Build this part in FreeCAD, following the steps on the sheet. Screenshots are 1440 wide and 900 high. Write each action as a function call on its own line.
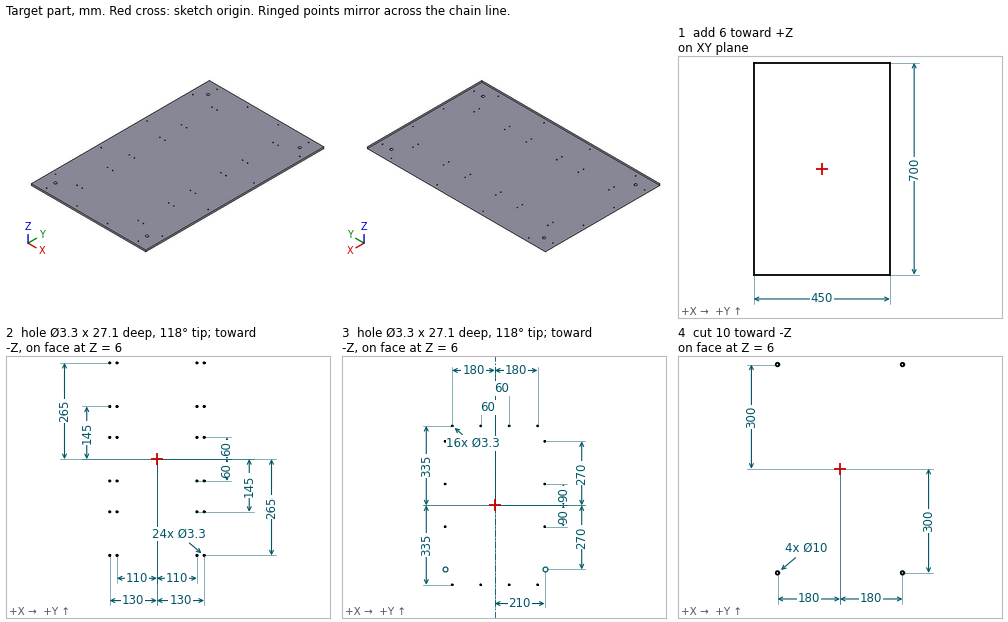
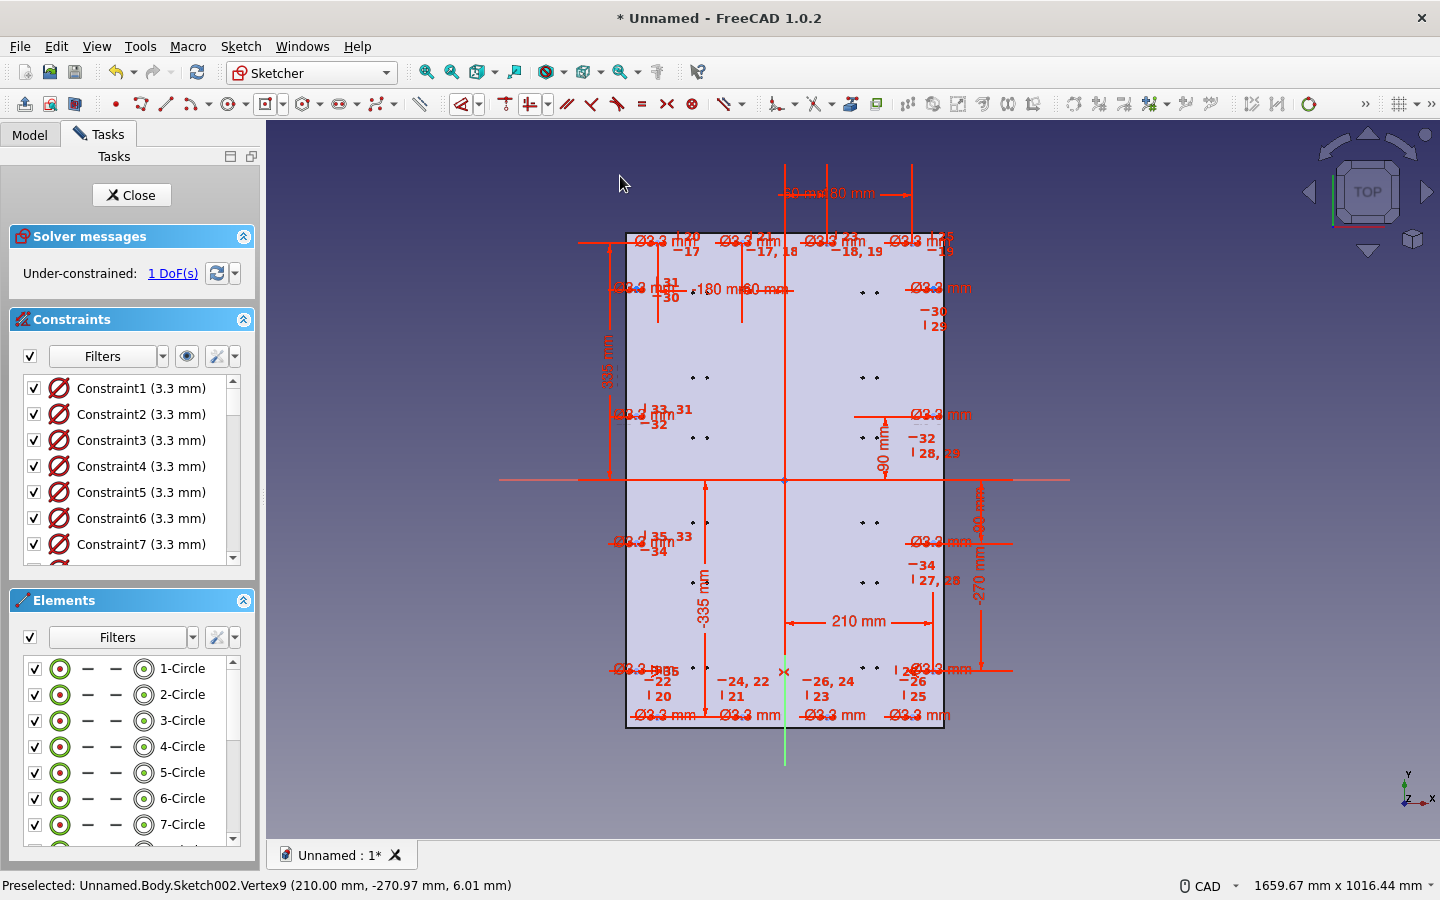
click(933, 290)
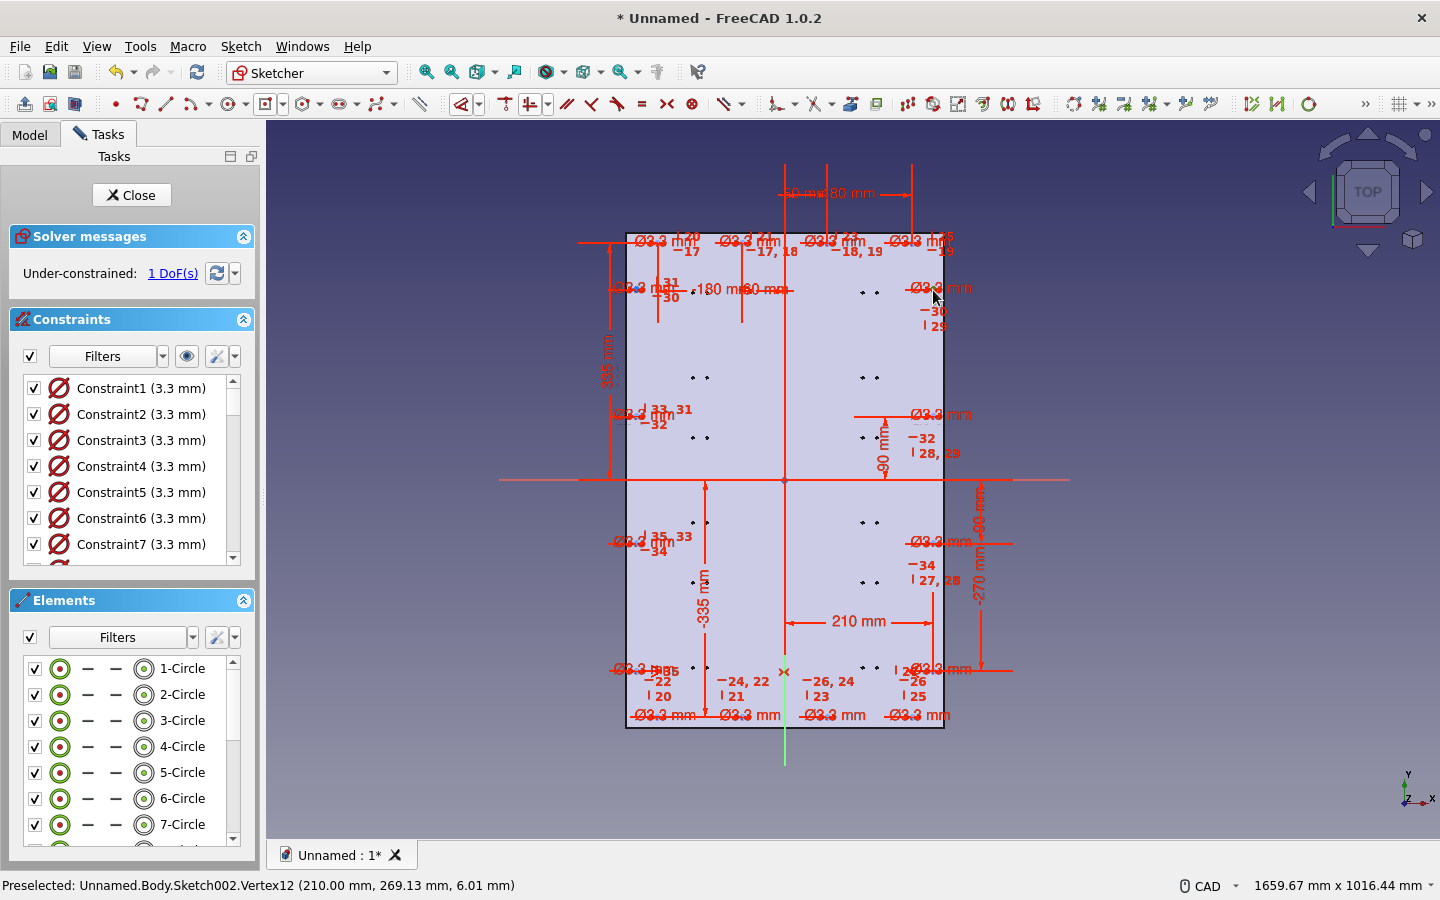
key(i)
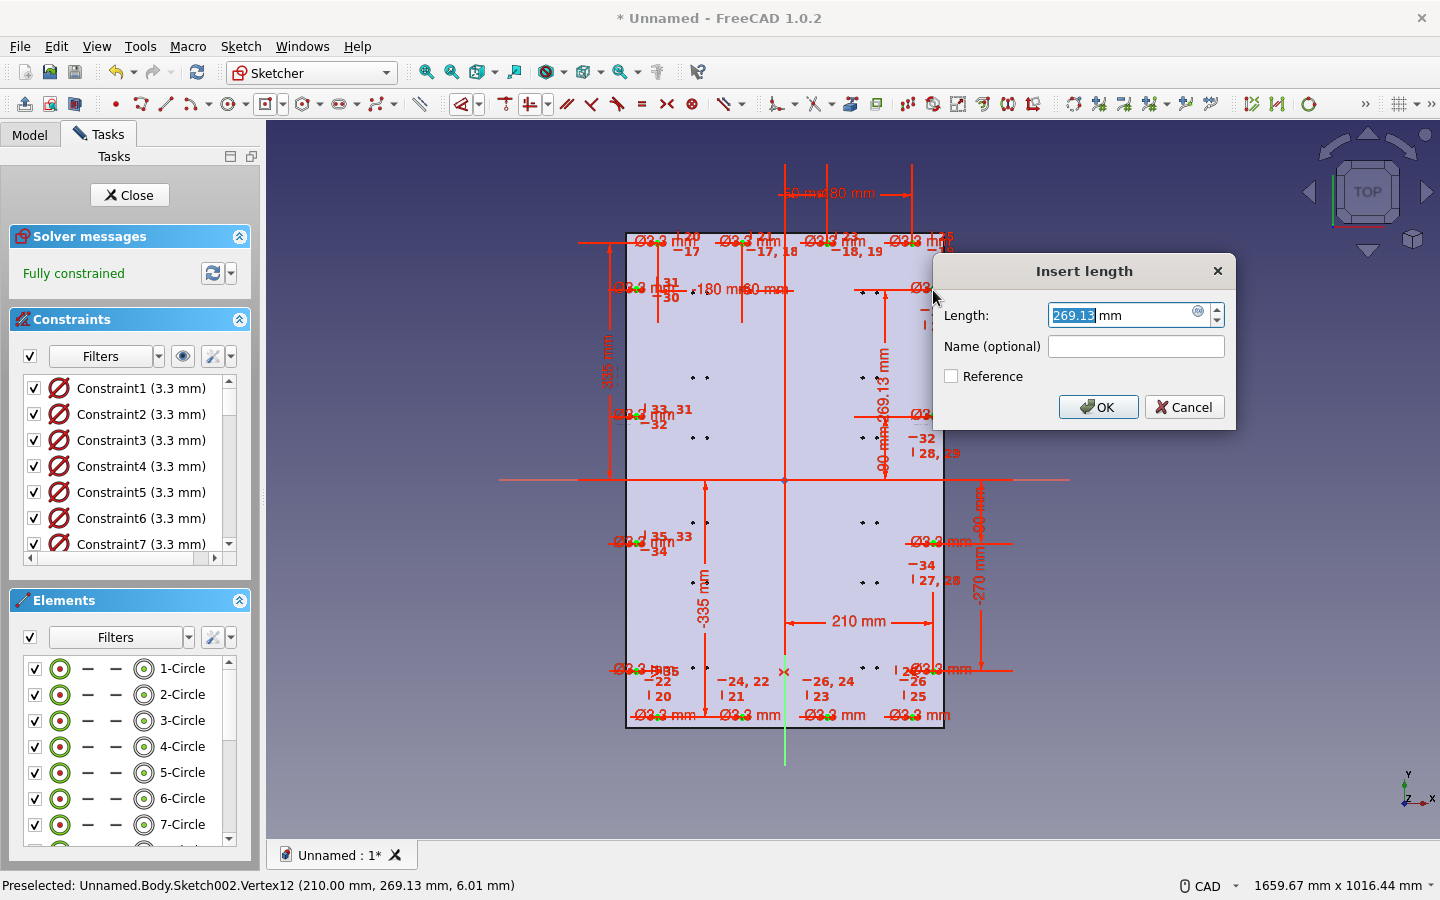
text(270)
key(Return)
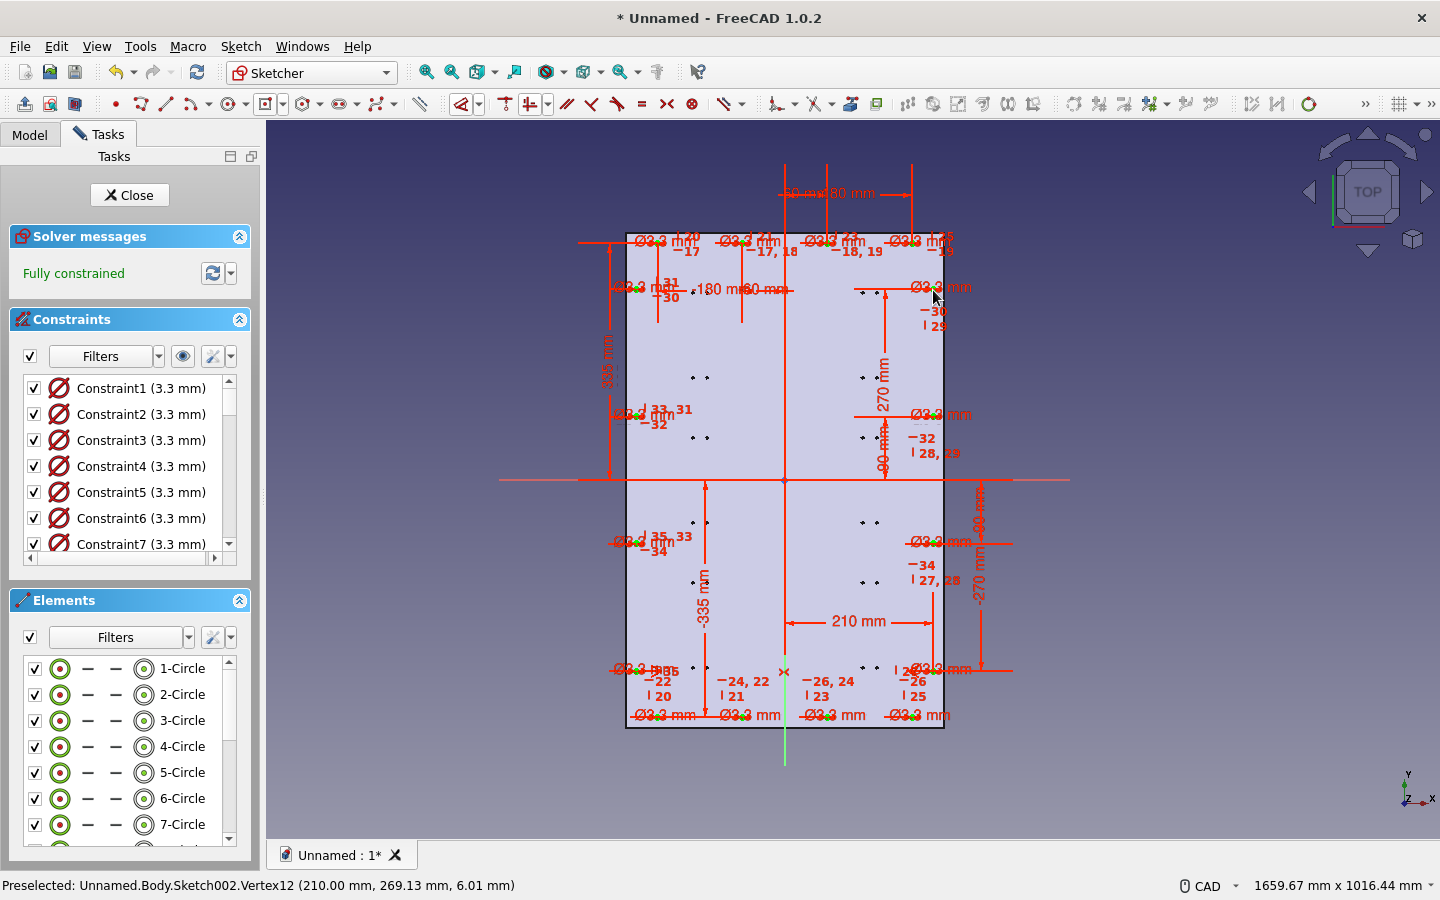
click(130, 195)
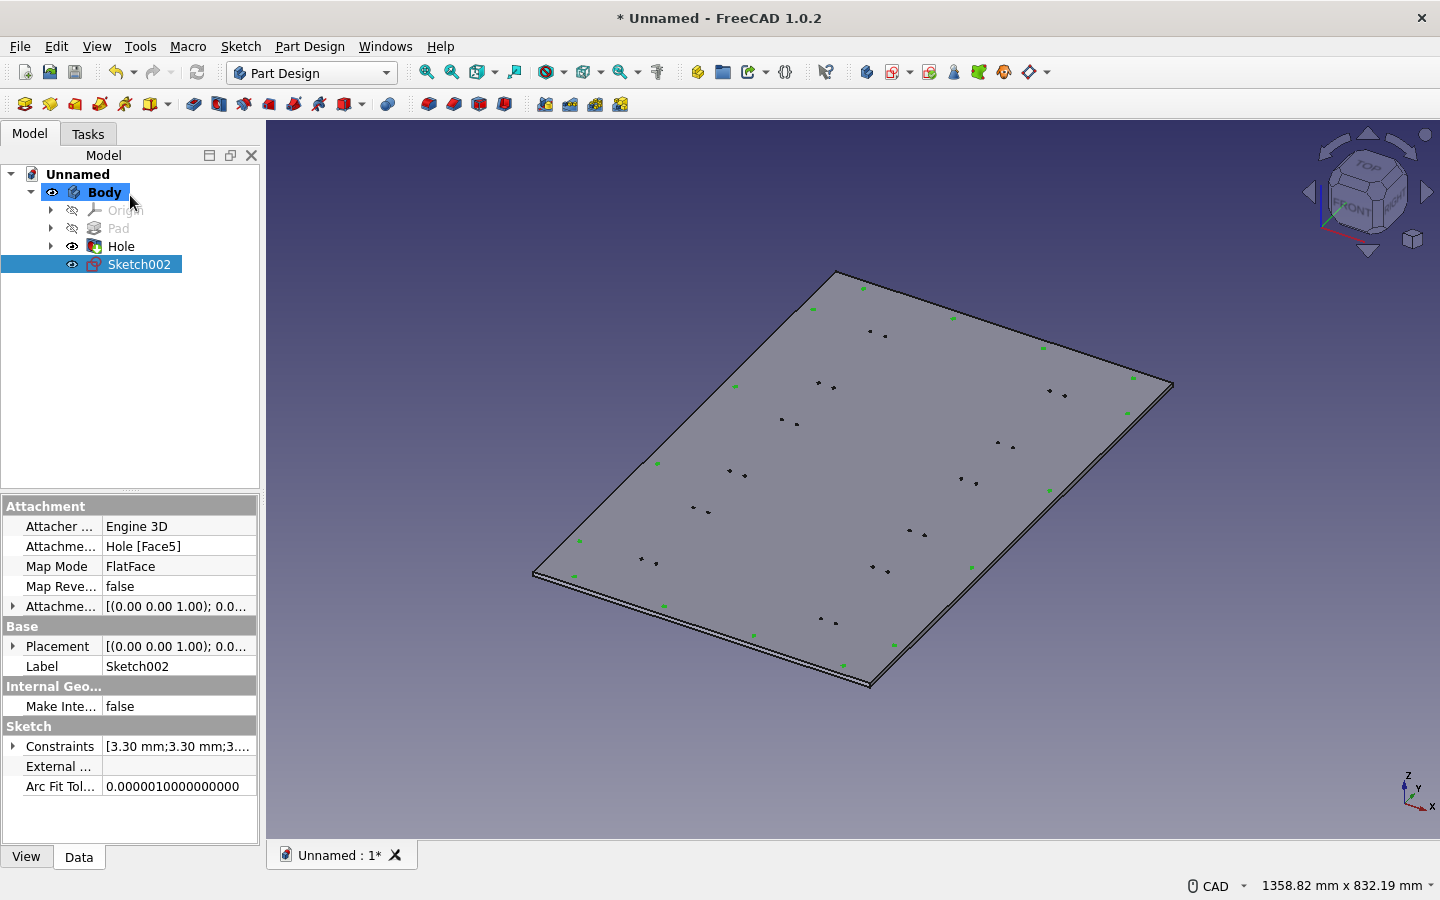
click(219, 104)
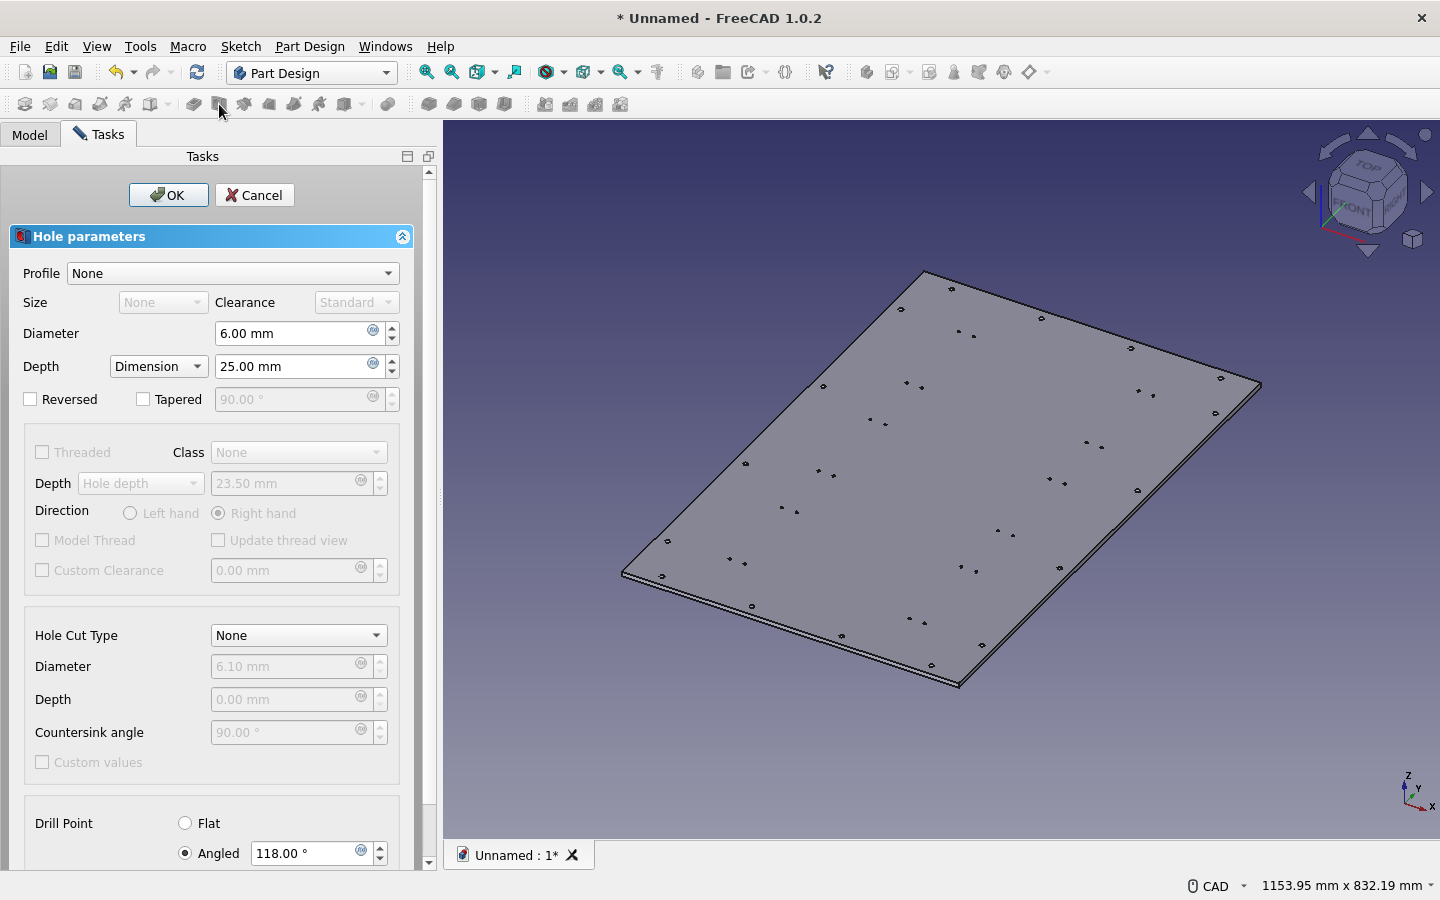
triple_click(300, 334)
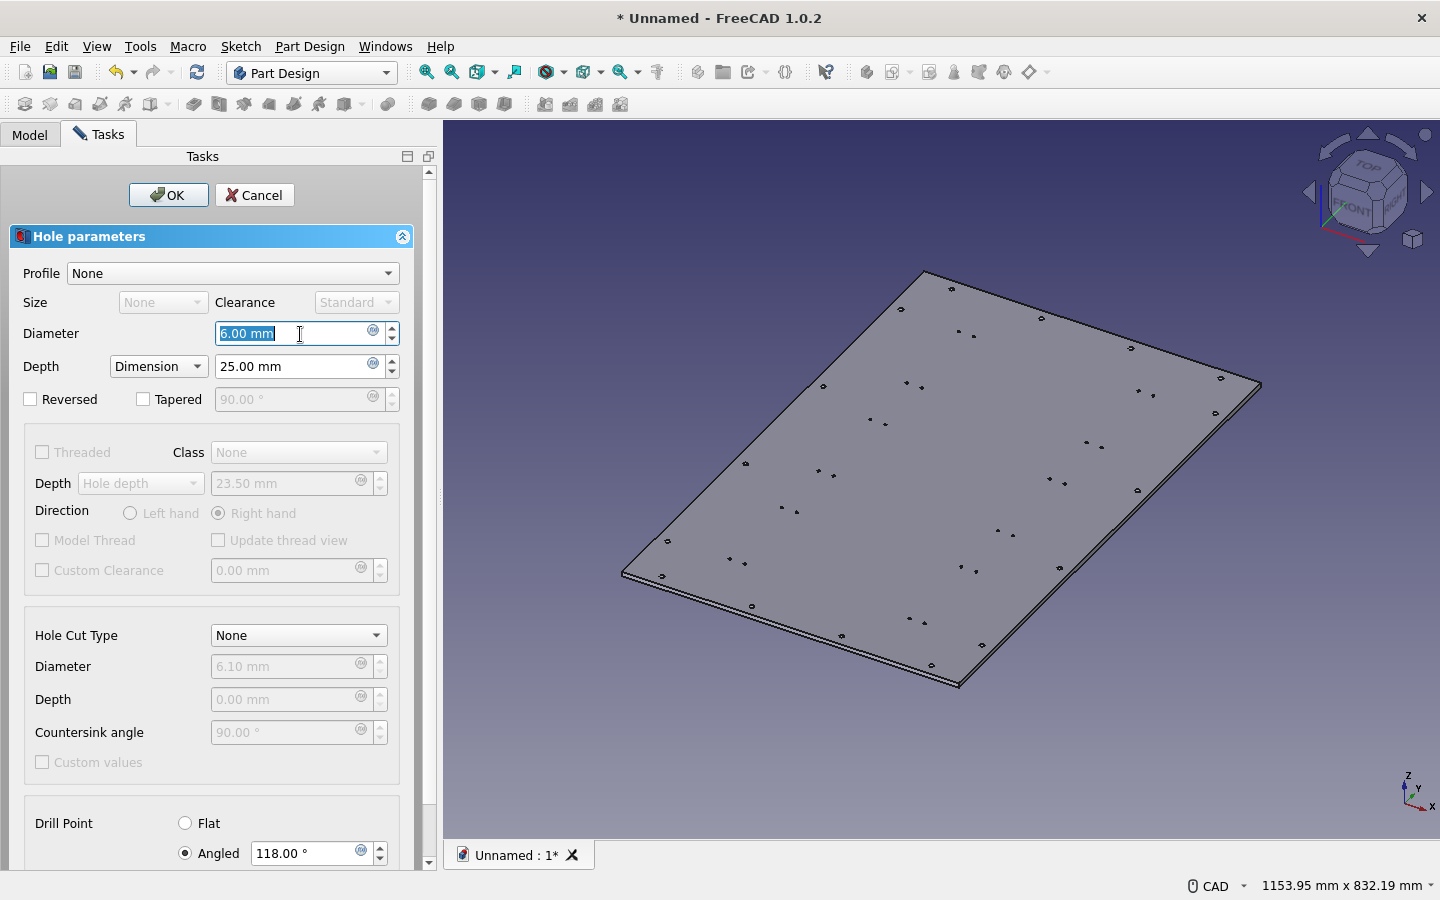
text(3.3)
key(Tab)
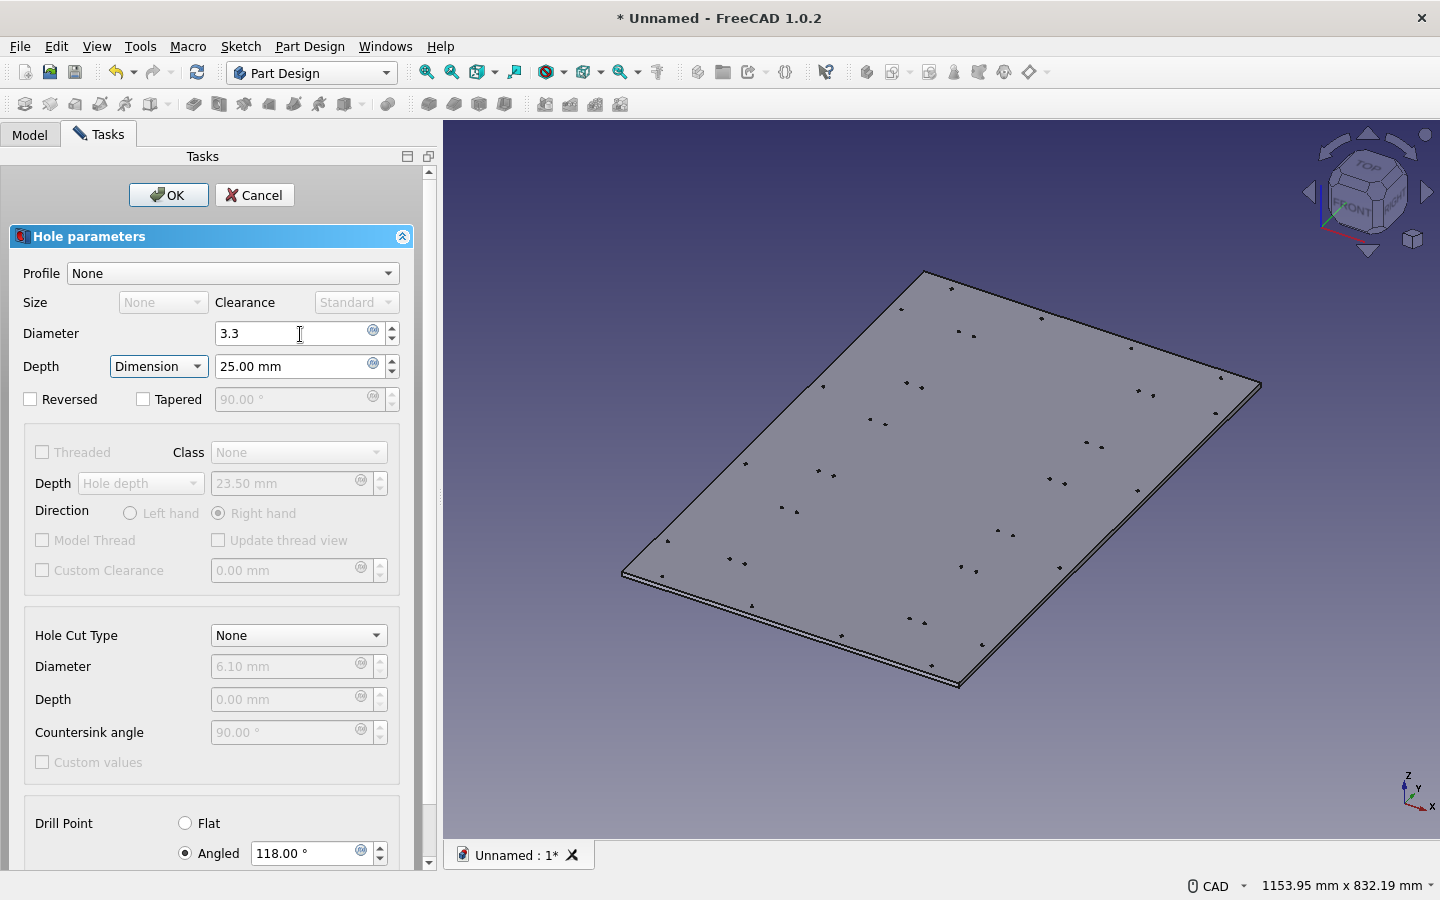
triple_click(300, 366)